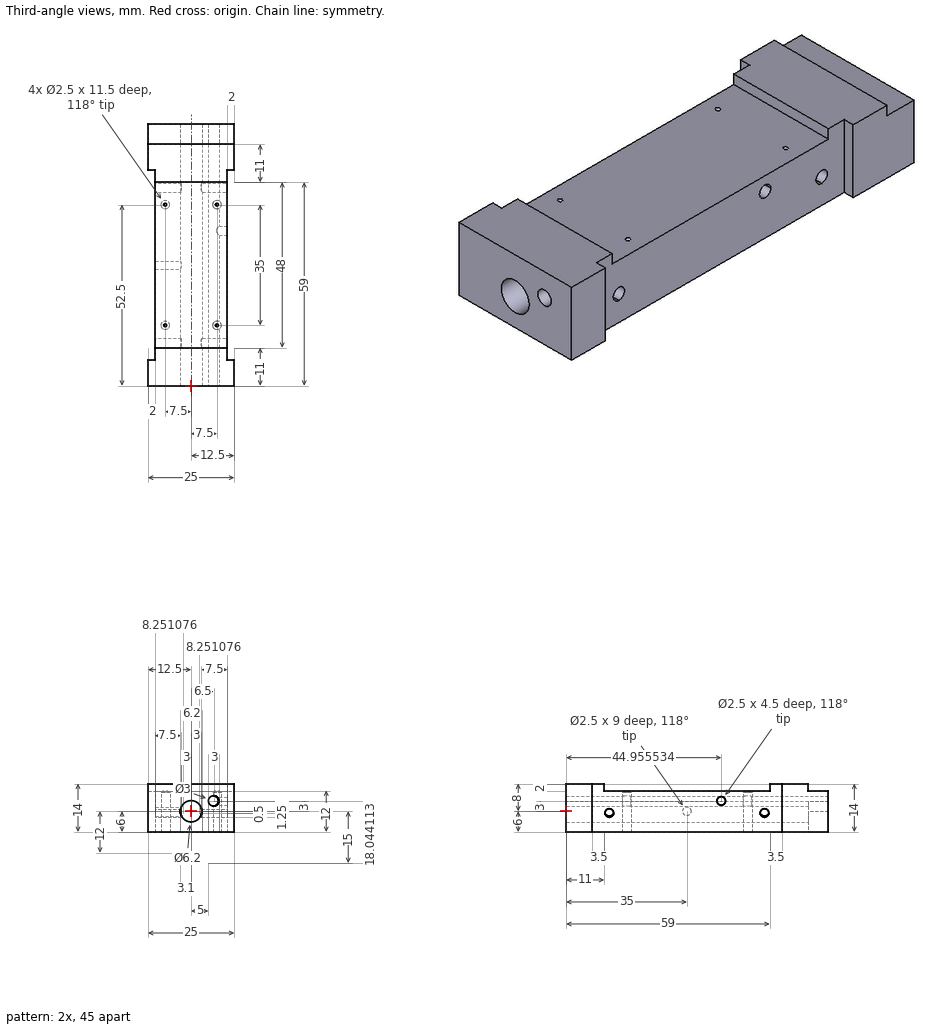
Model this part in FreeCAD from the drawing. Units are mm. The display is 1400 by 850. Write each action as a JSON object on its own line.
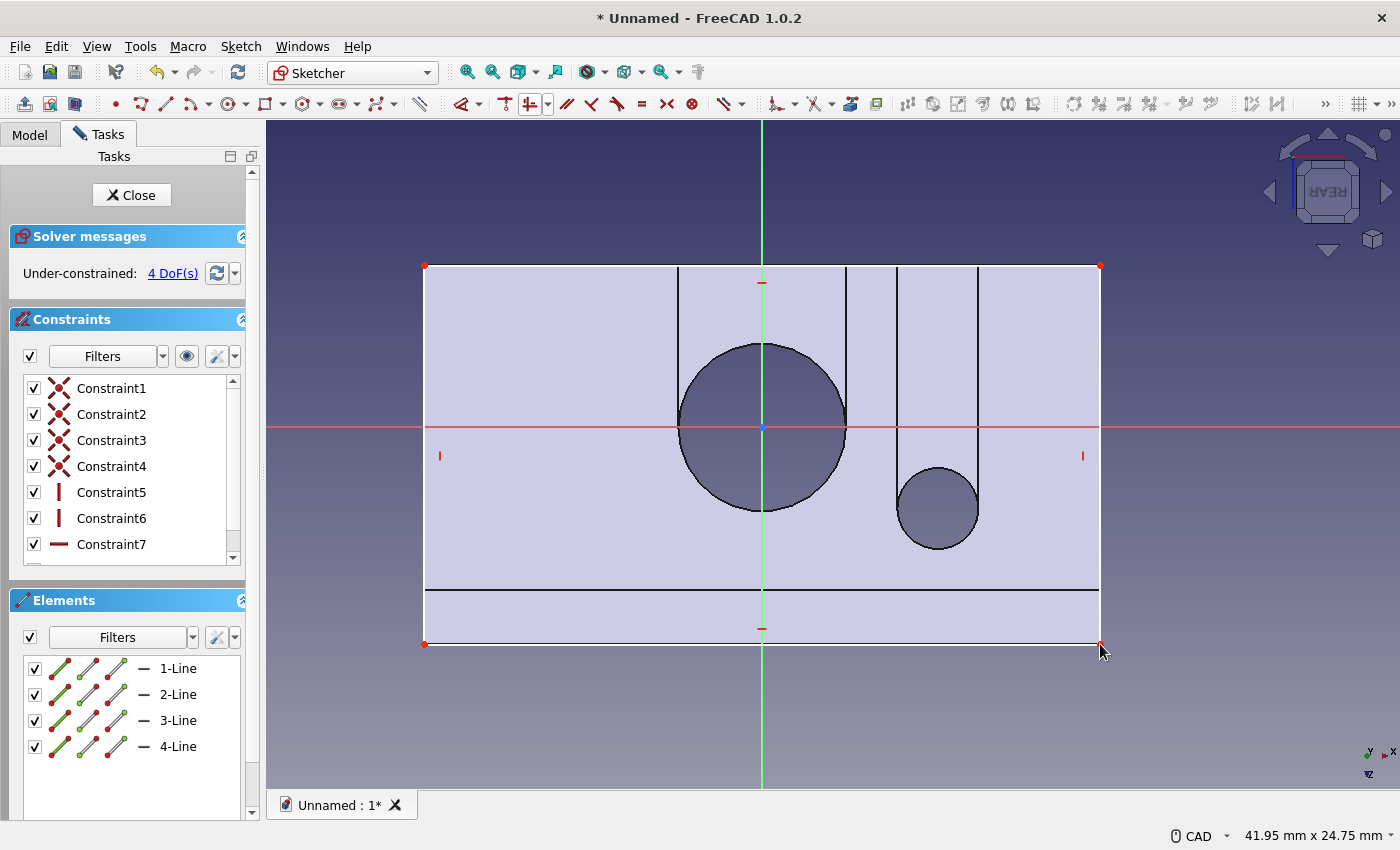
{"action": "left_click", "coordinate": [460, 104]}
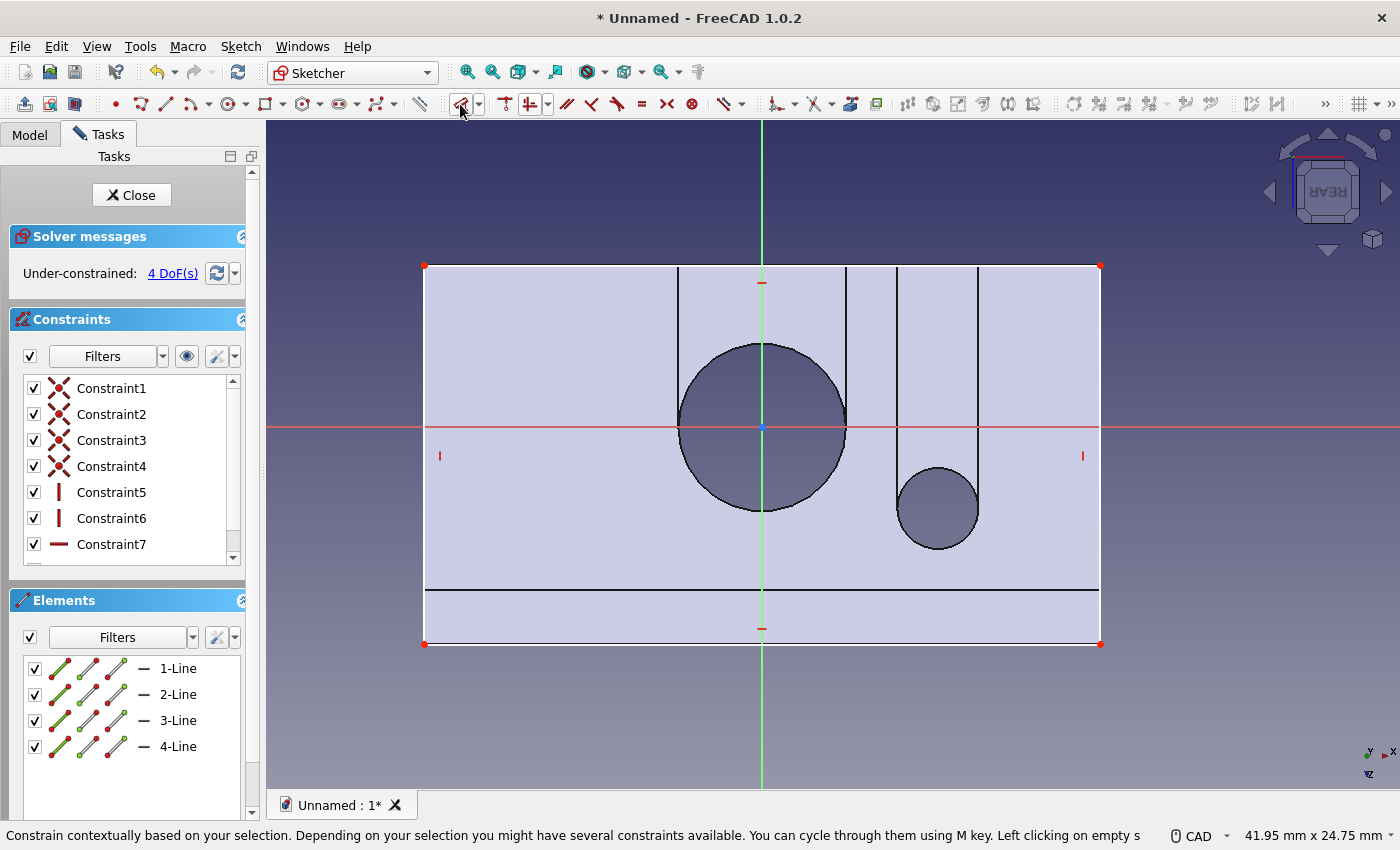
{"action": "left_click", "coordinate": [424, 380]}
{"action": "left_click", "coordinate": [390, 455]}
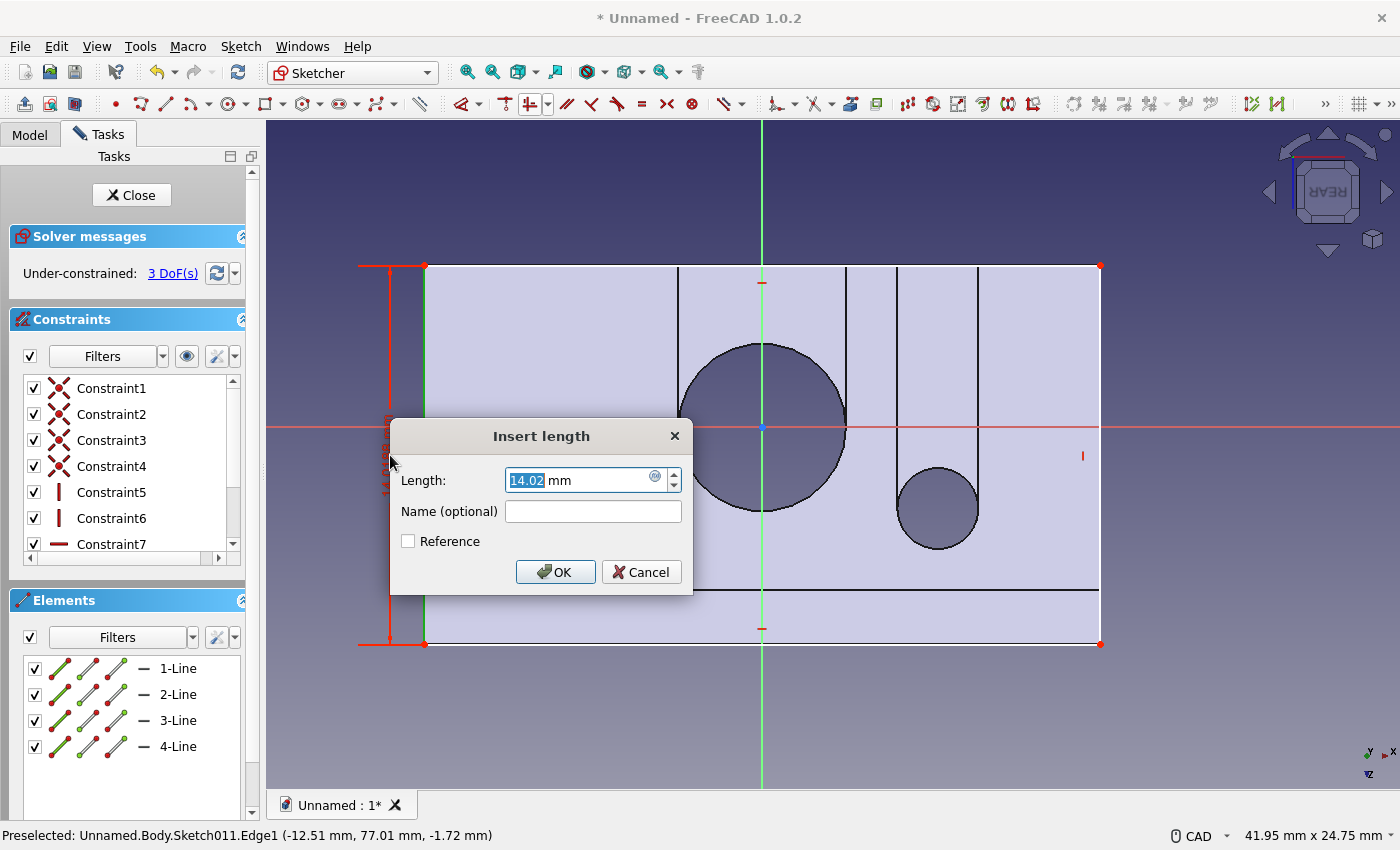
{"action": "type", "text": "14"}
{"action": "key", "text": "Return"}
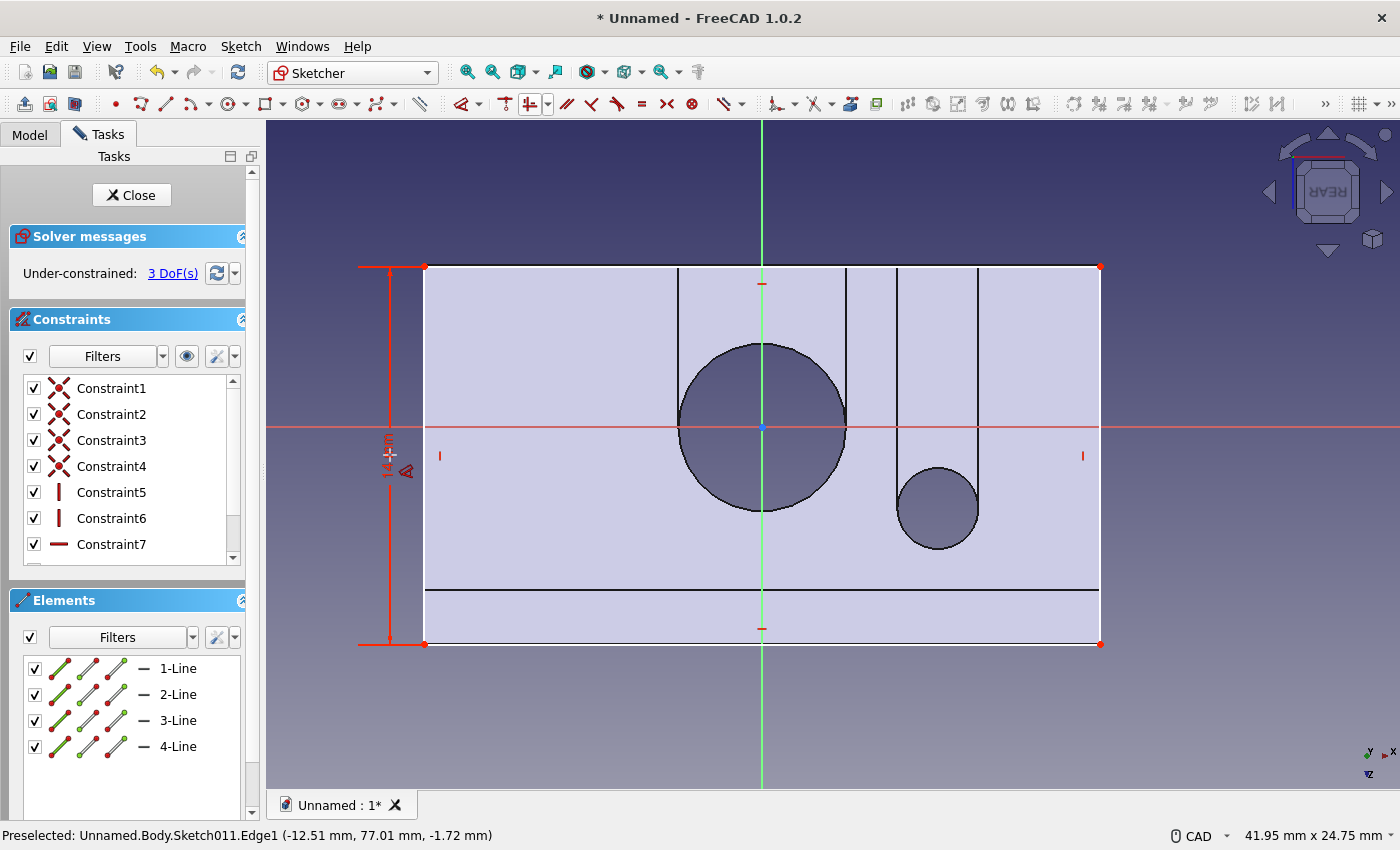
{"action": "left_click", "coordinate": [627, 645]}
{"action": "left_click", "coordinate": [607, 679]}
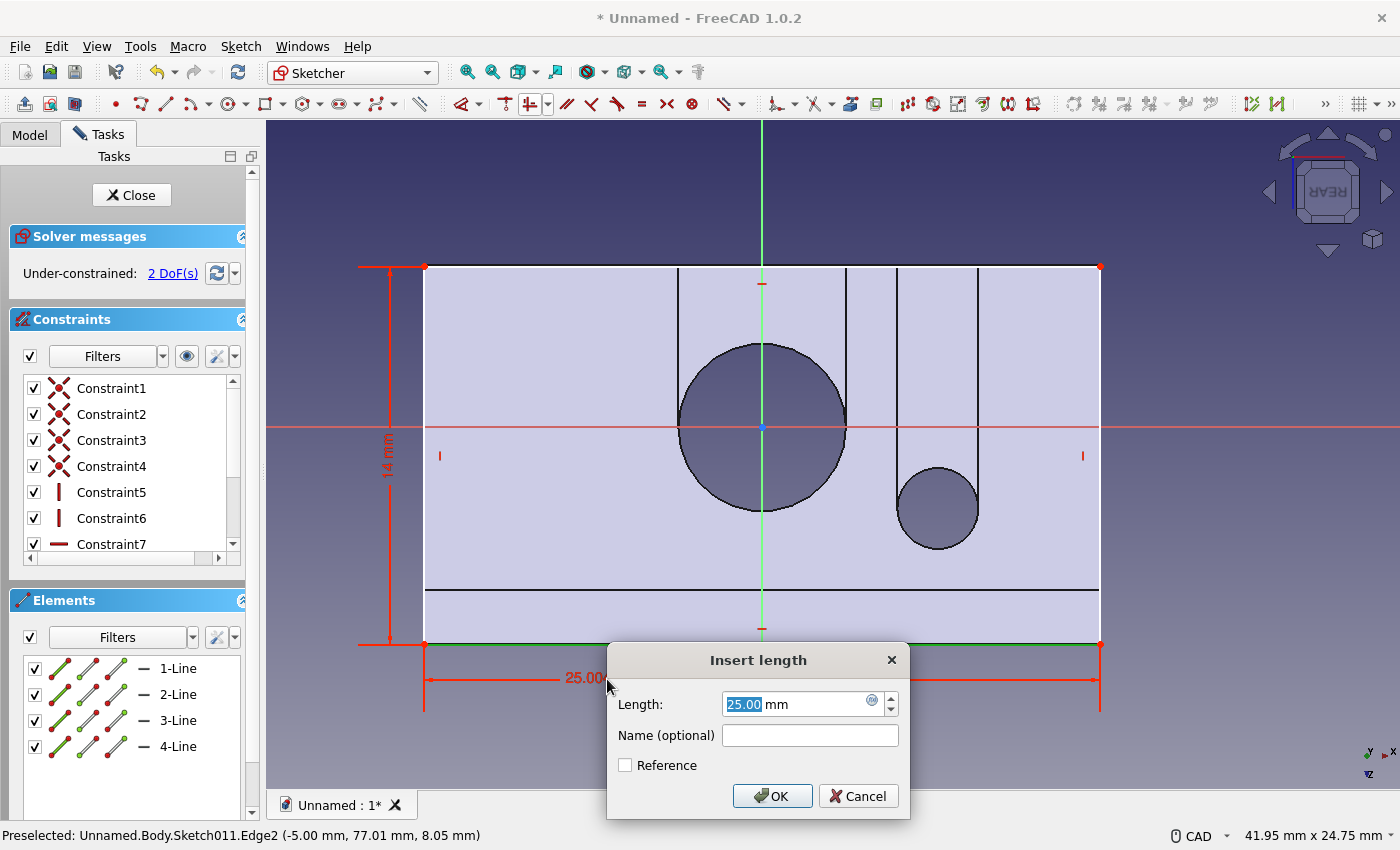
{"action": "type", "text": "25"}
{"action": "key", "text": "Return"}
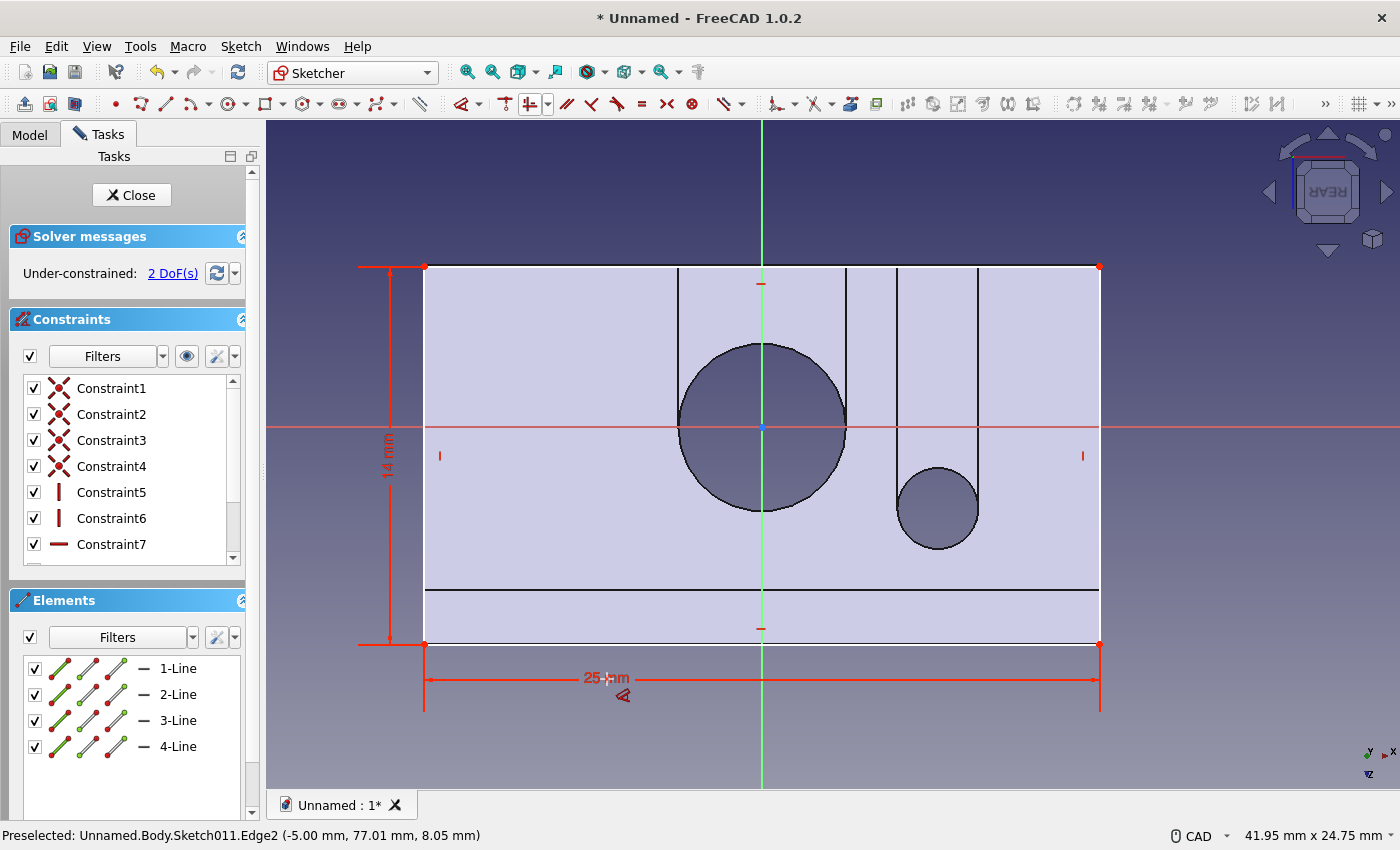
{"action": "left_click", "coordinate": [424, 267]}
{"action": "left_click", "coordinate": [390, 347]}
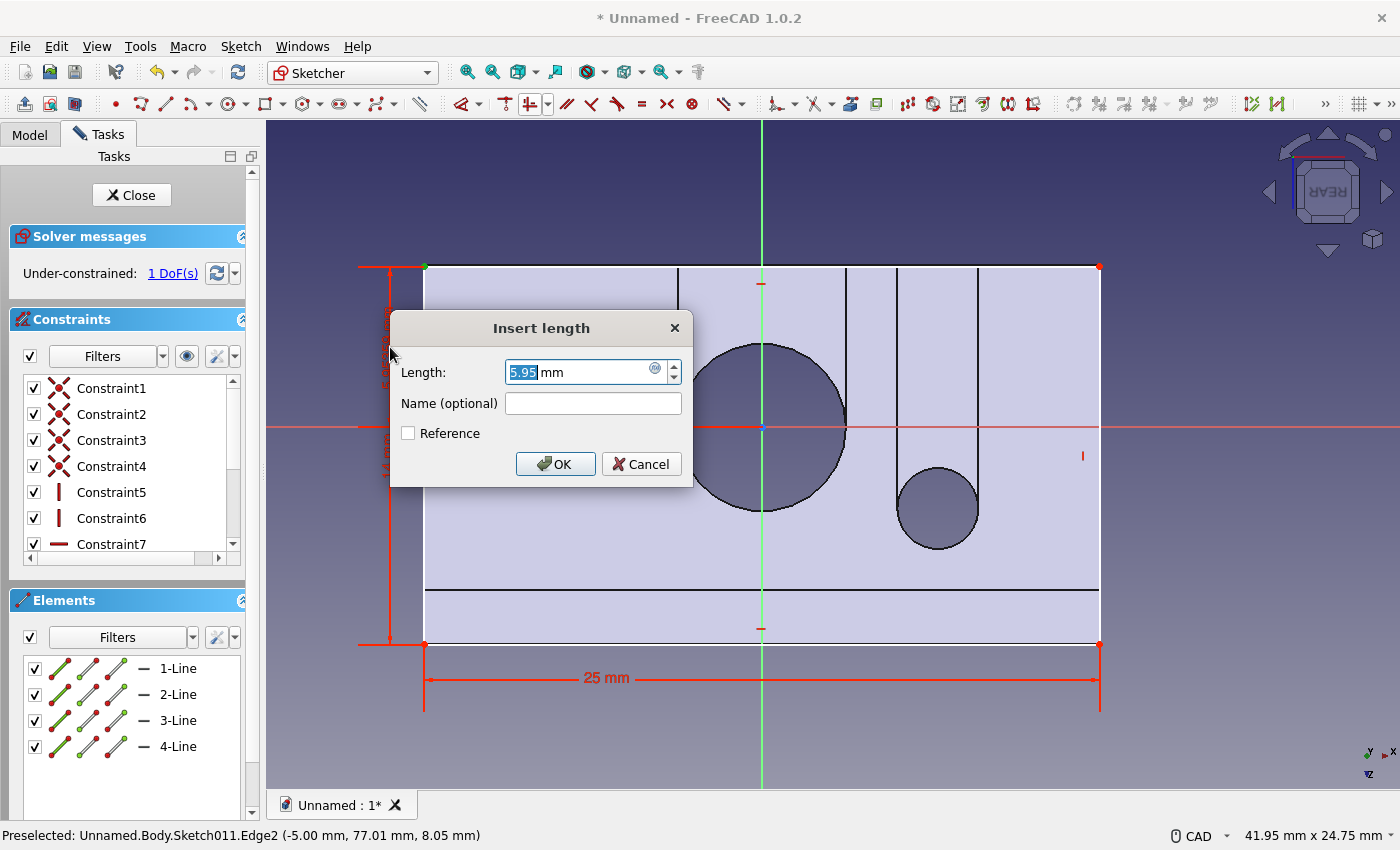
{"action": "type", "text": "6"}
{"action": "key", "text": "Return"}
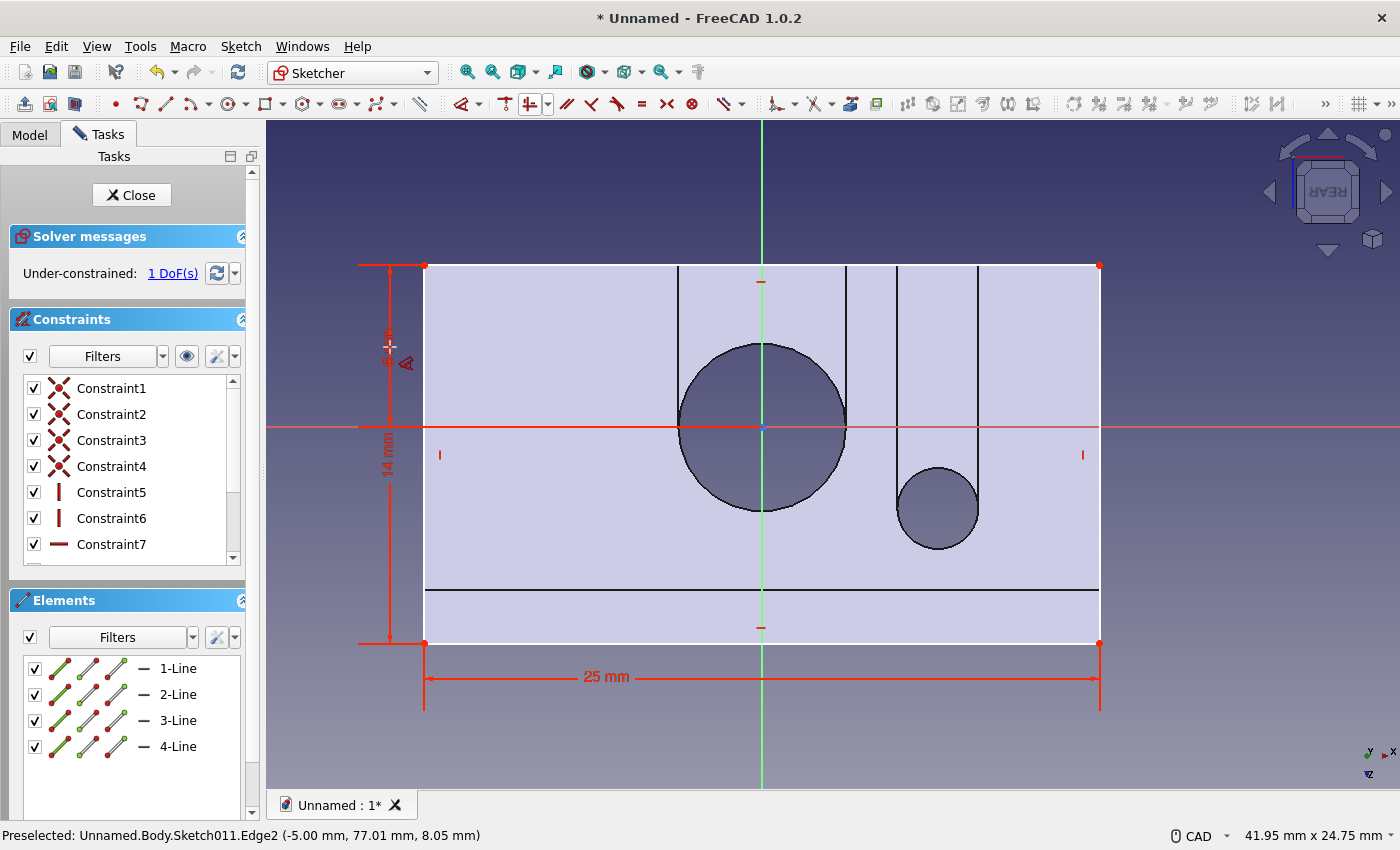
{"action": "left_click", "coordinate": [424, 265]}
{"action": "left_click", "coordinate": [593, 231]}